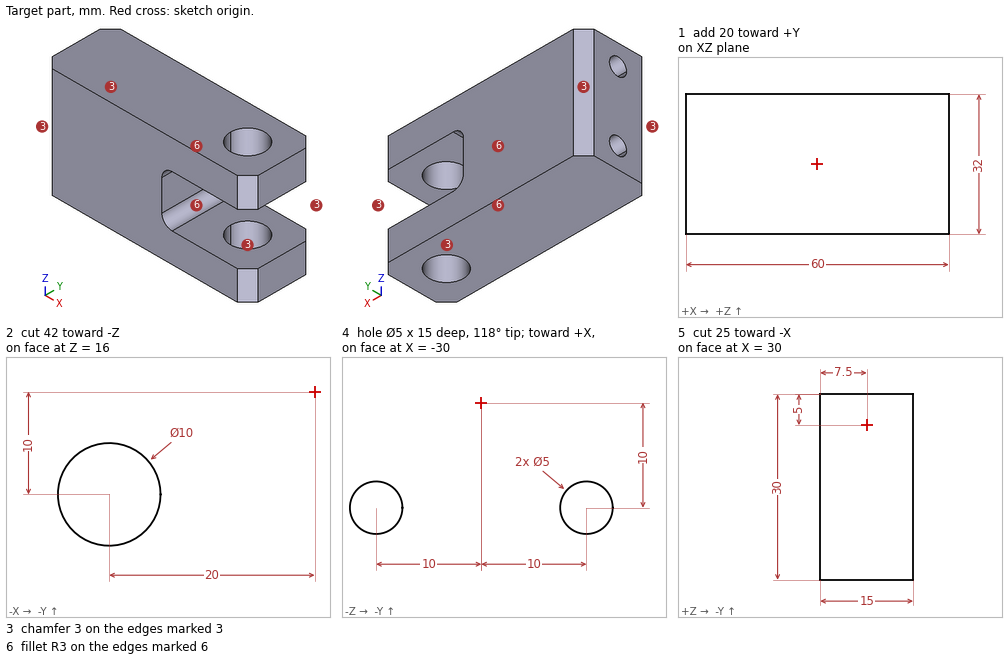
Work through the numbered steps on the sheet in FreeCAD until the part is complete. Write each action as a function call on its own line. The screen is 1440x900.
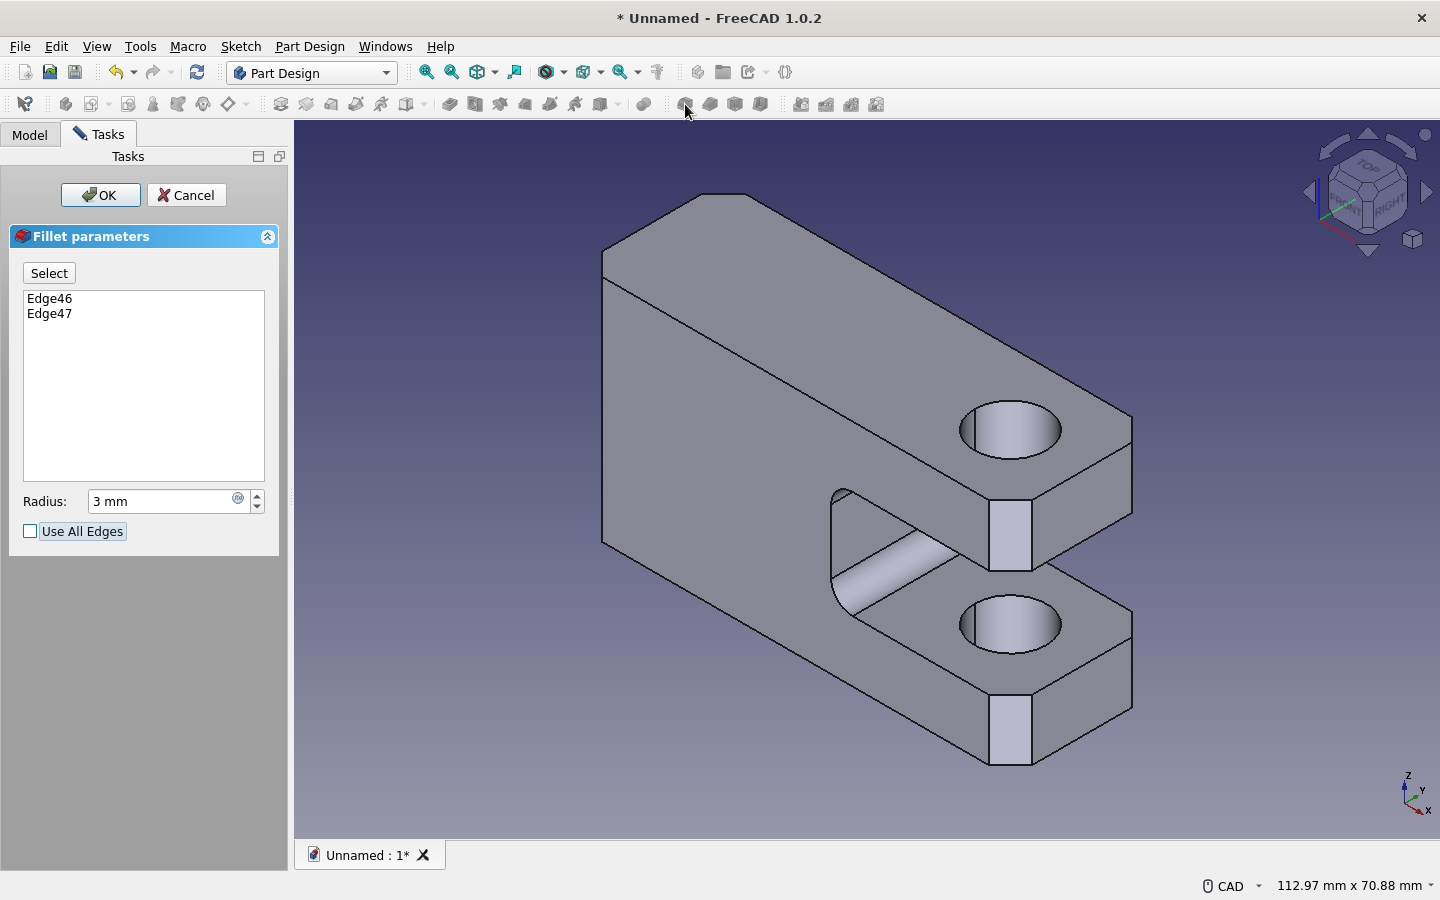
click(101, 195)